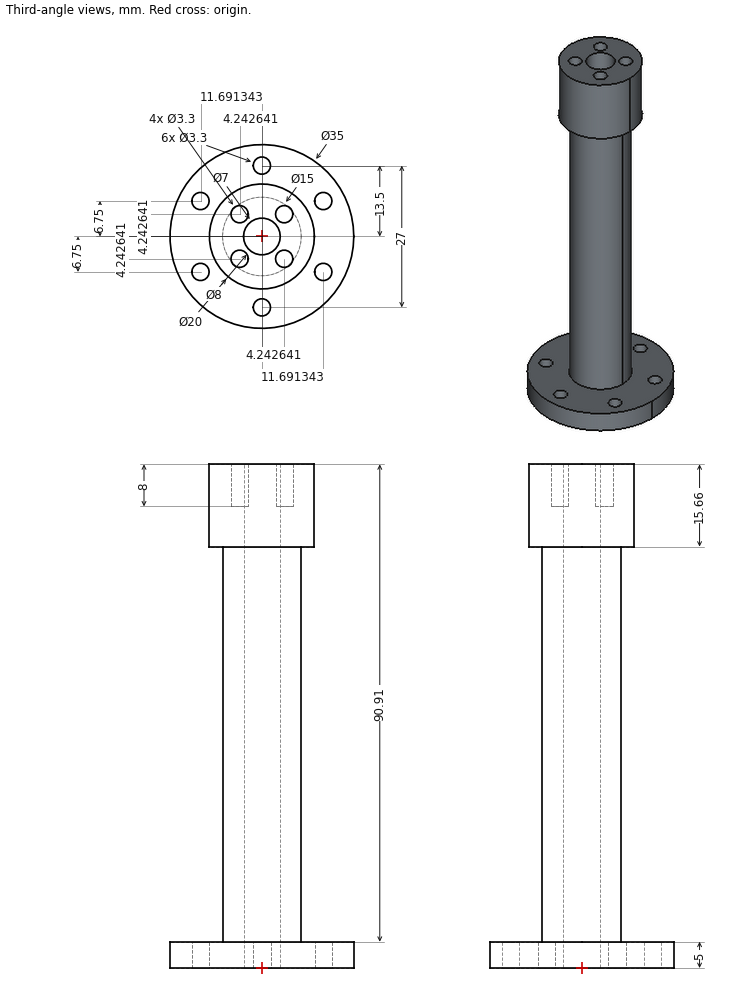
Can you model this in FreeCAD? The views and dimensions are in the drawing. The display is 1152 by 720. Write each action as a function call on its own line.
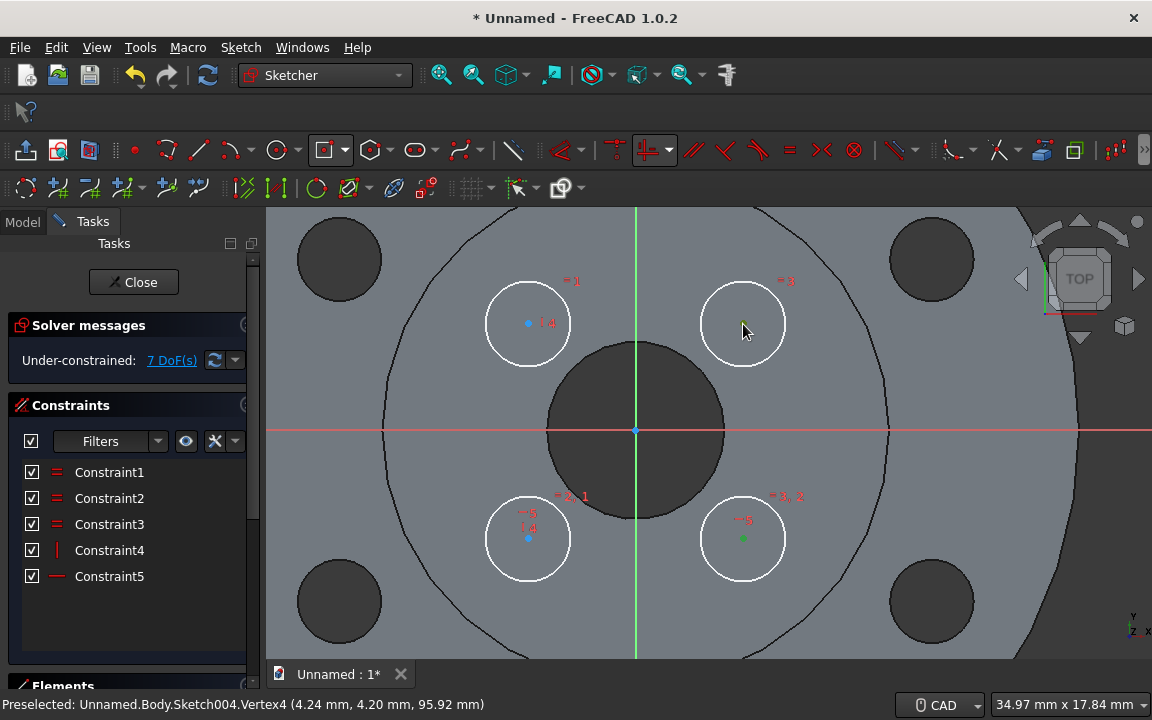
key(v)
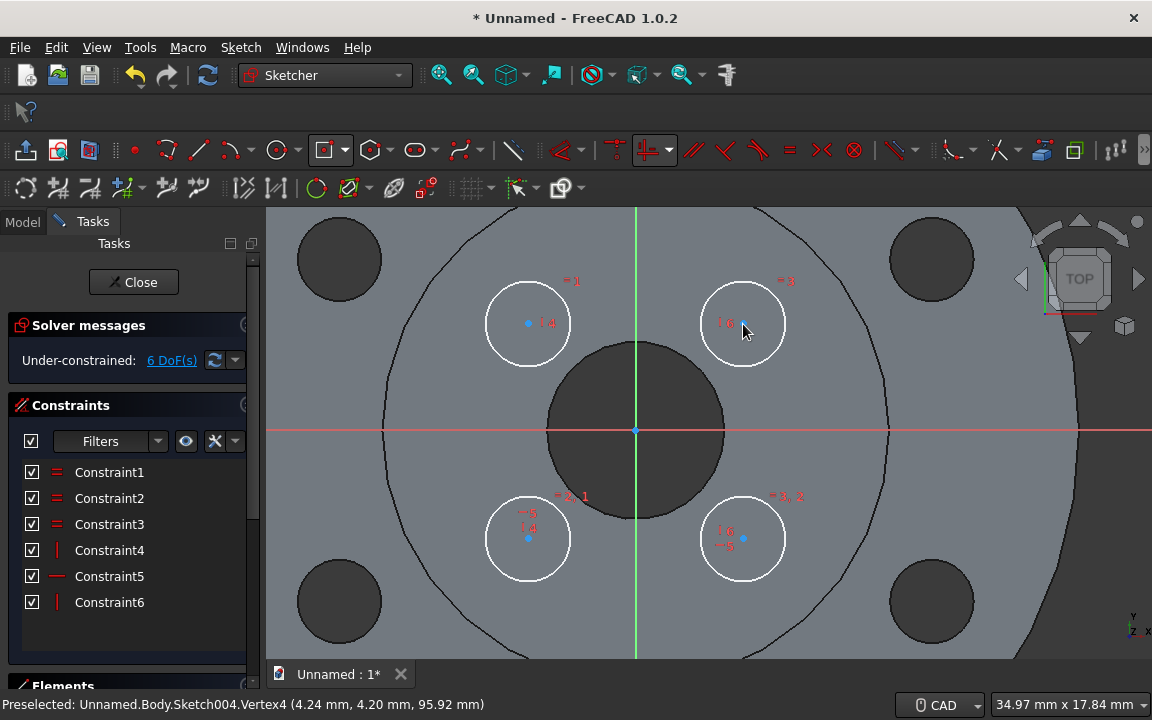
click(528, 324)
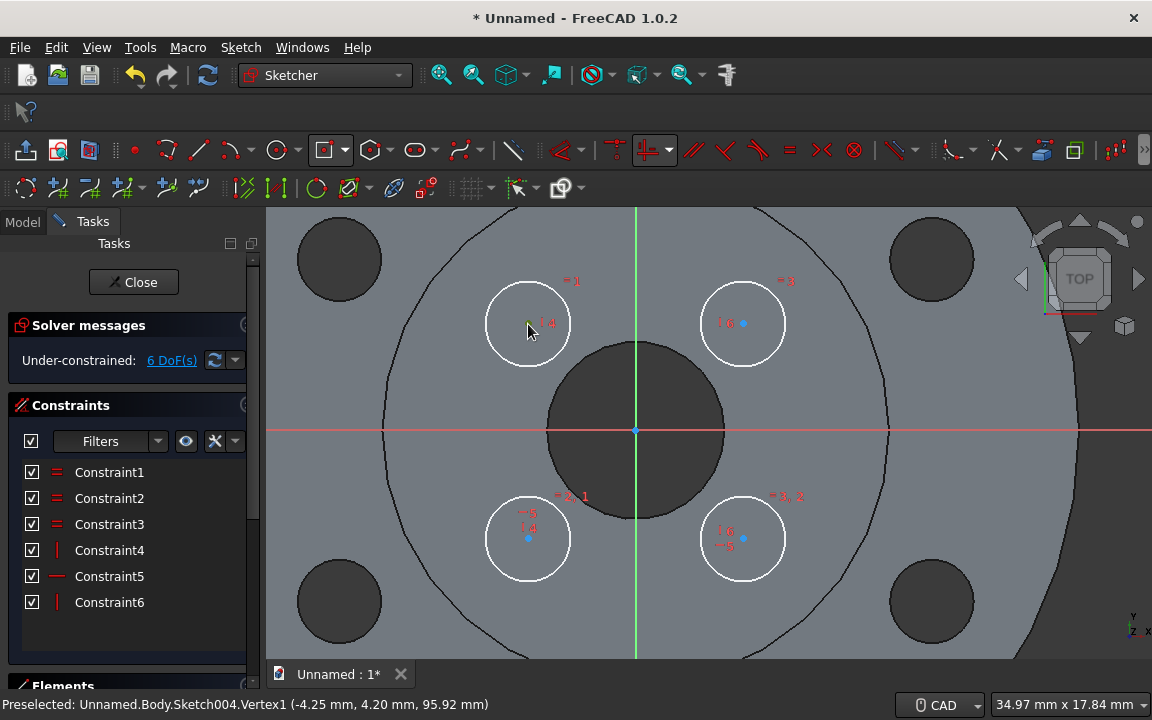
click(743, 324)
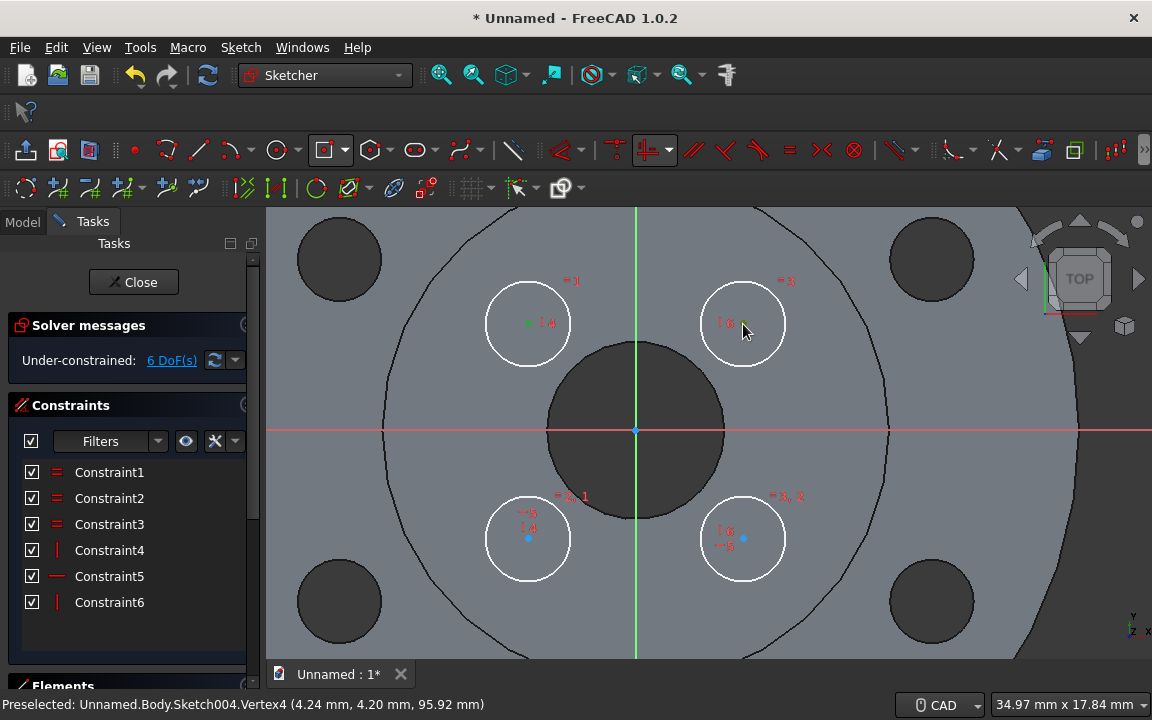
key(h)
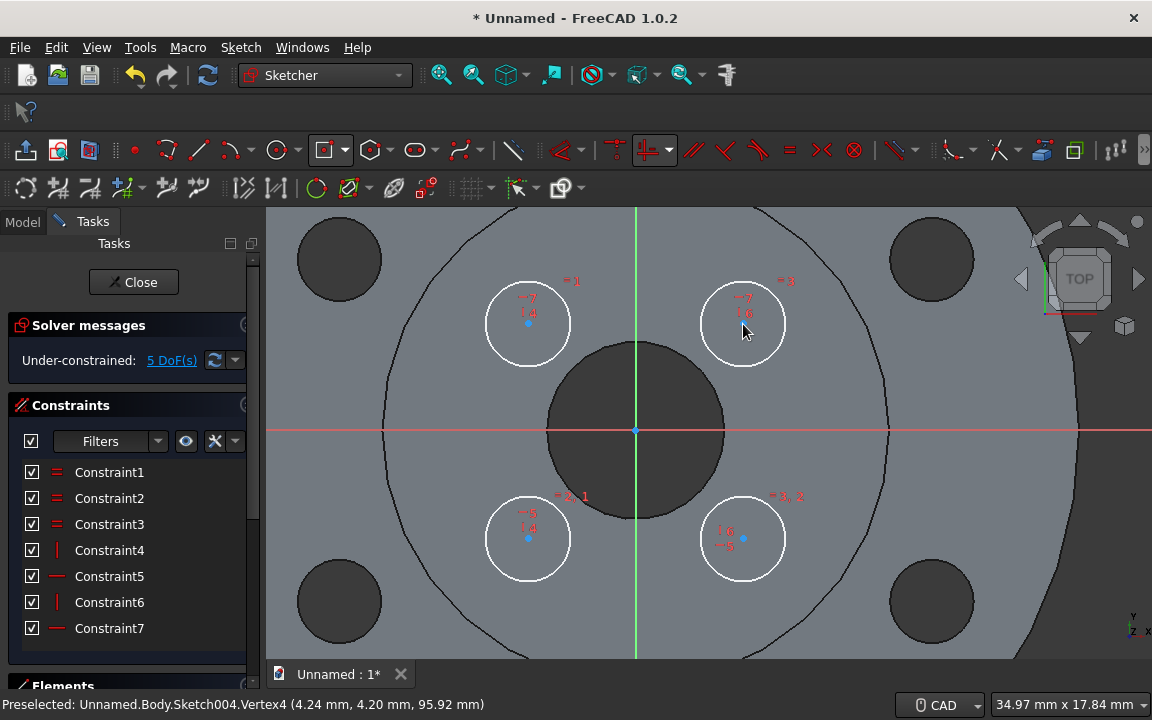
key(d)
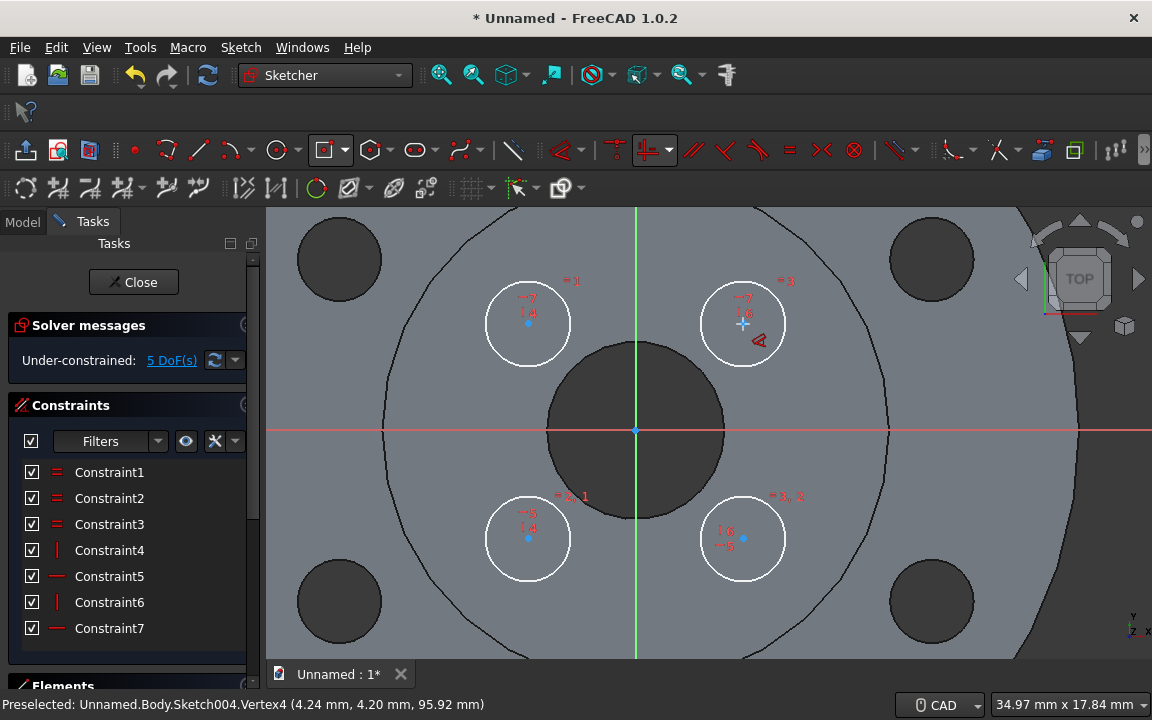
click(558, 294)
click(581, 271)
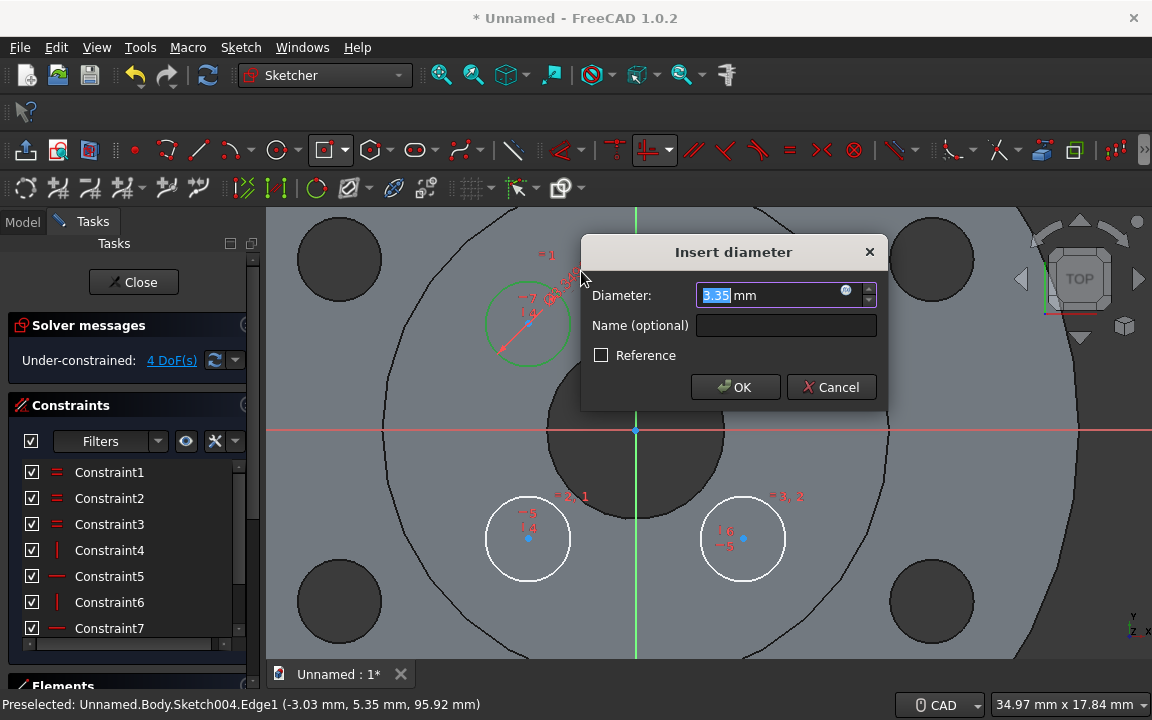
text(3.3)
key(Return)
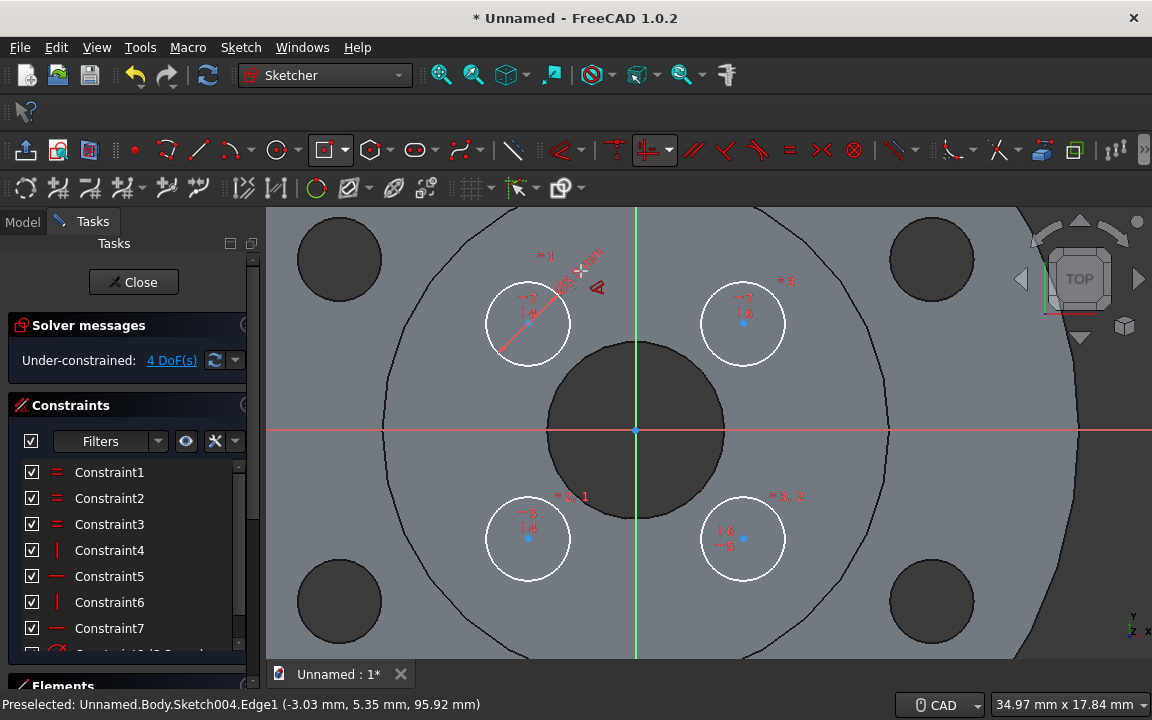
click(528, 324)
click(582, 464)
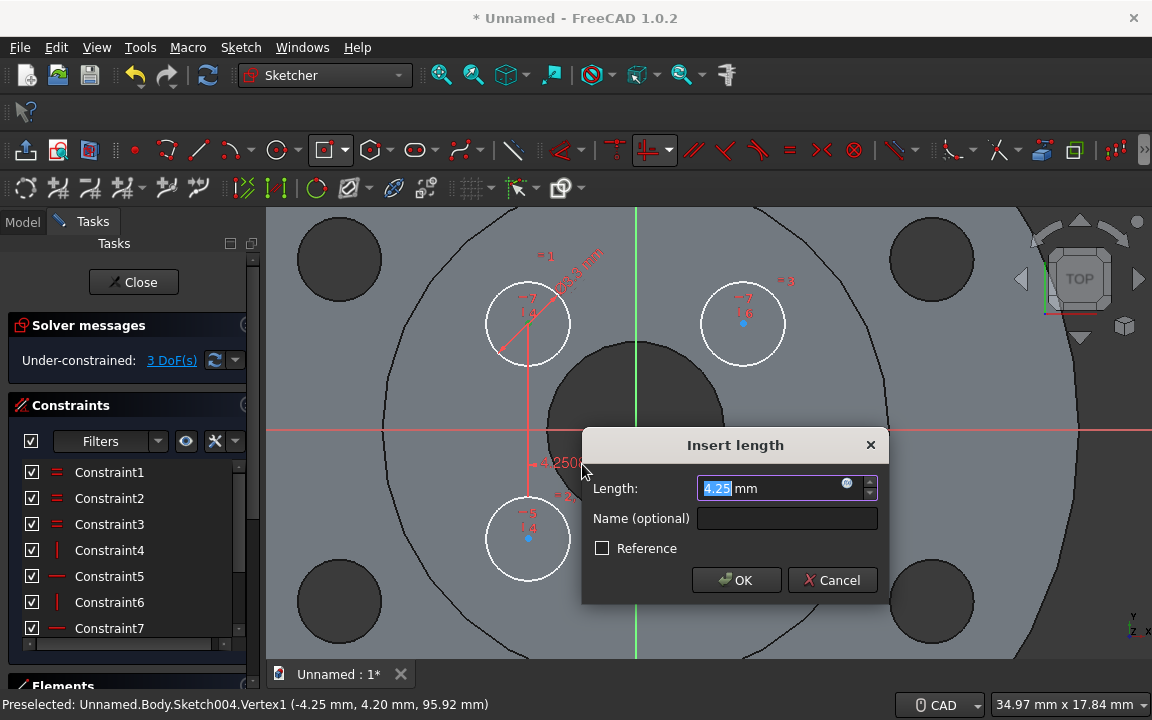
text(4.242641)
key(Return)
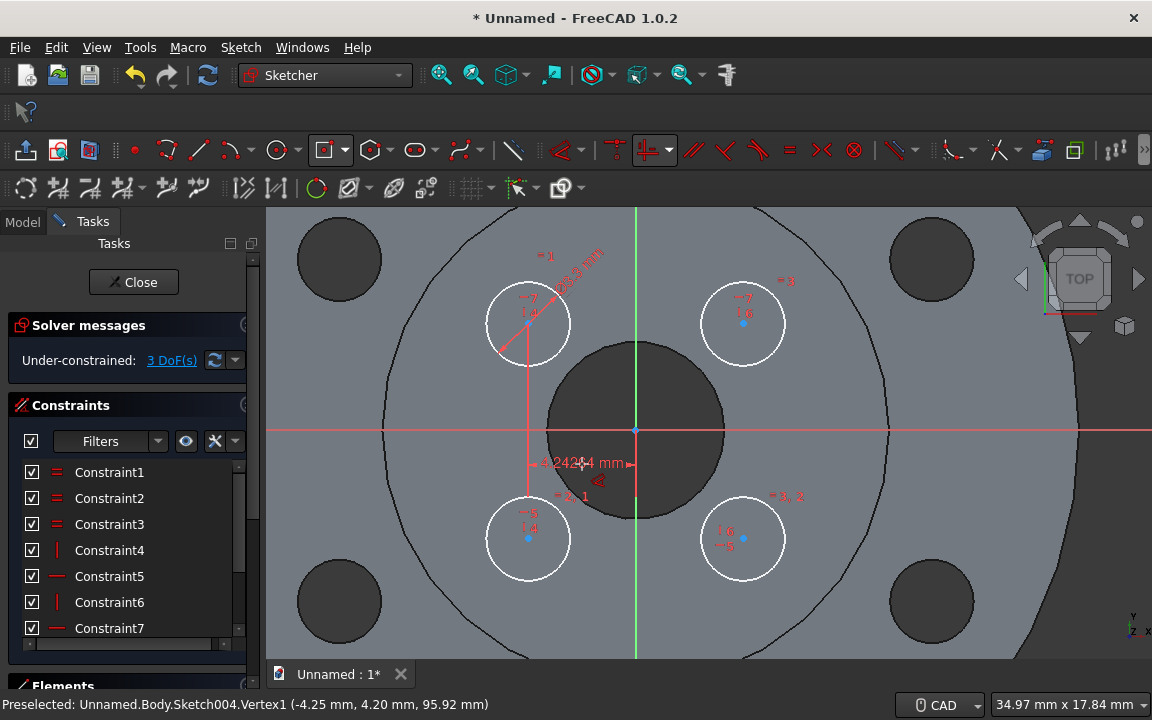
click(528, 324)
click(494, 377)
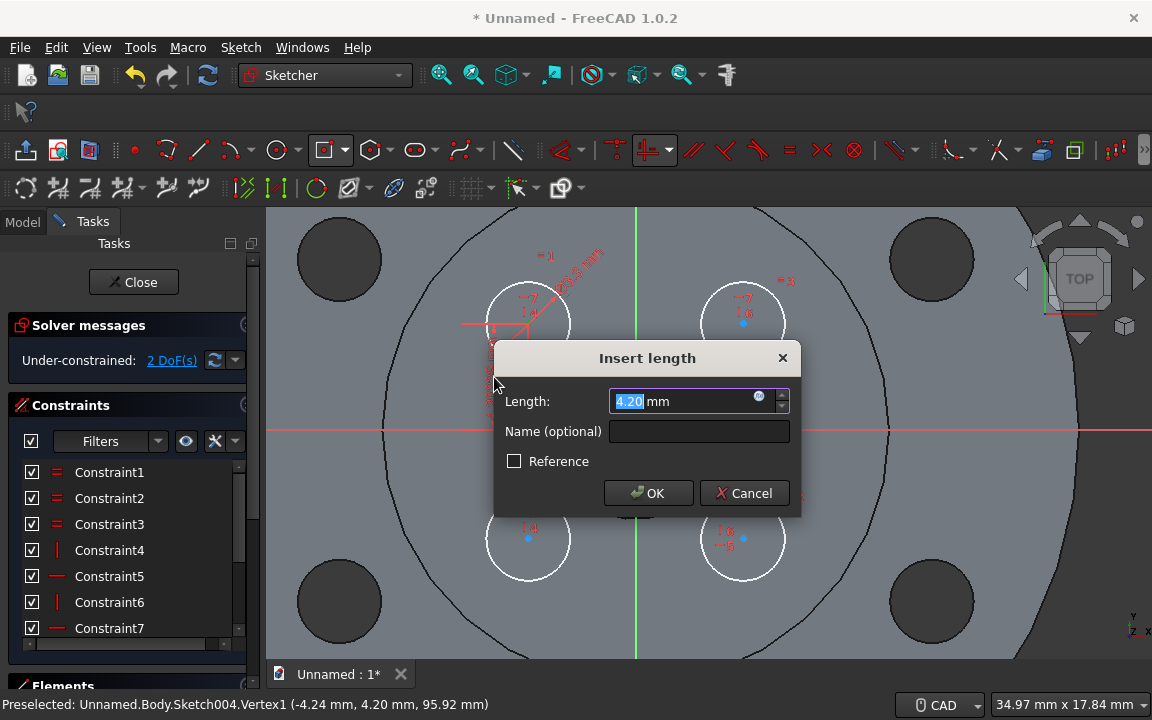
text(4.242641)
key(Return)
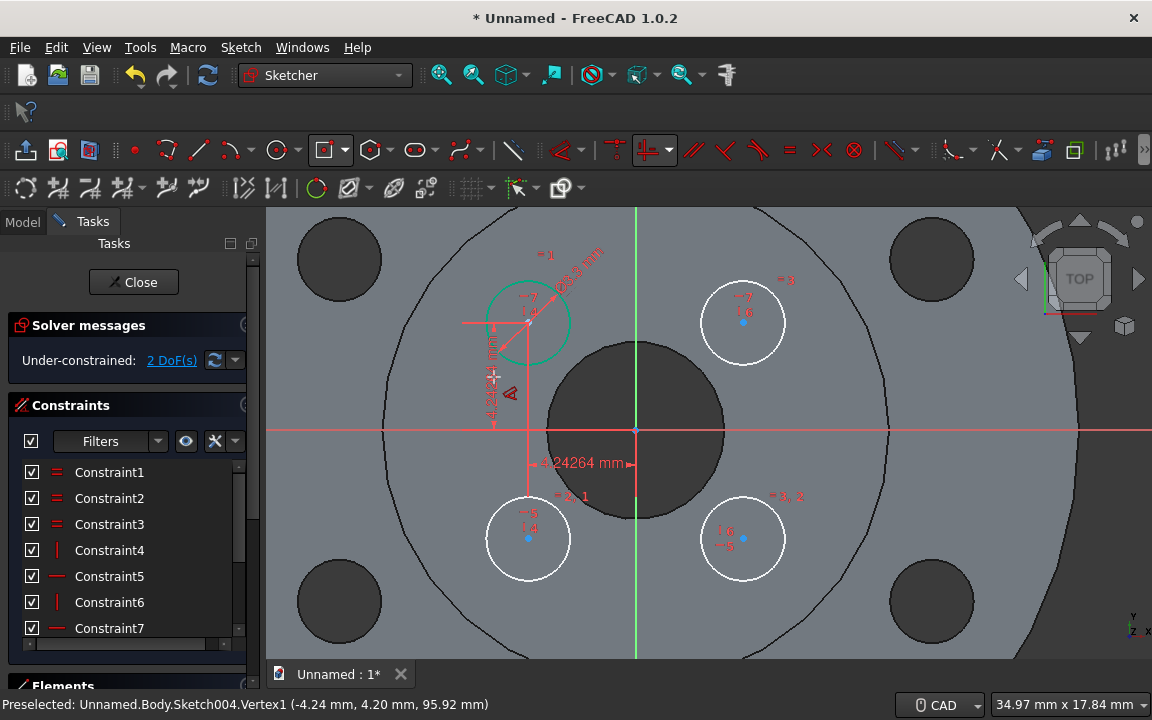
click(528, 539)
click(494, 485)